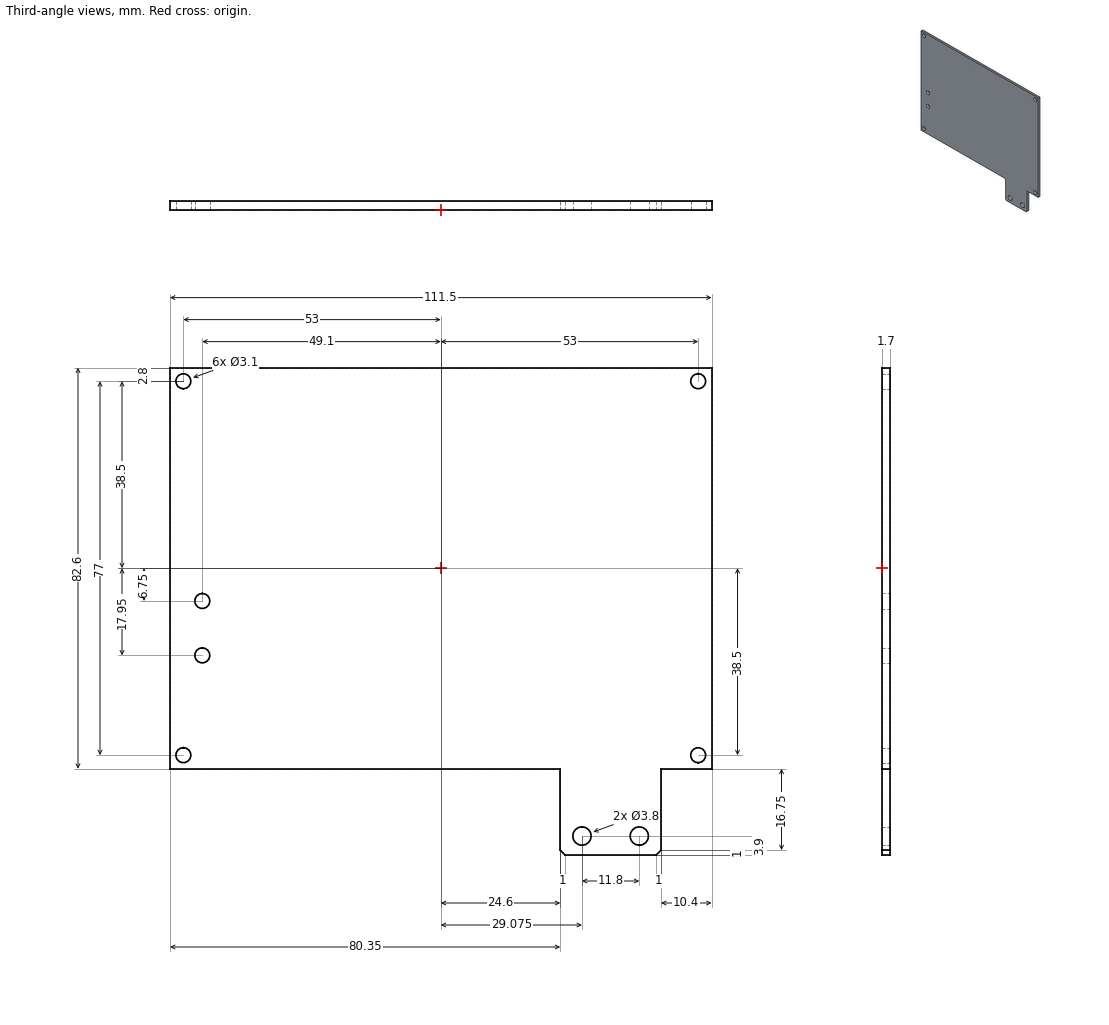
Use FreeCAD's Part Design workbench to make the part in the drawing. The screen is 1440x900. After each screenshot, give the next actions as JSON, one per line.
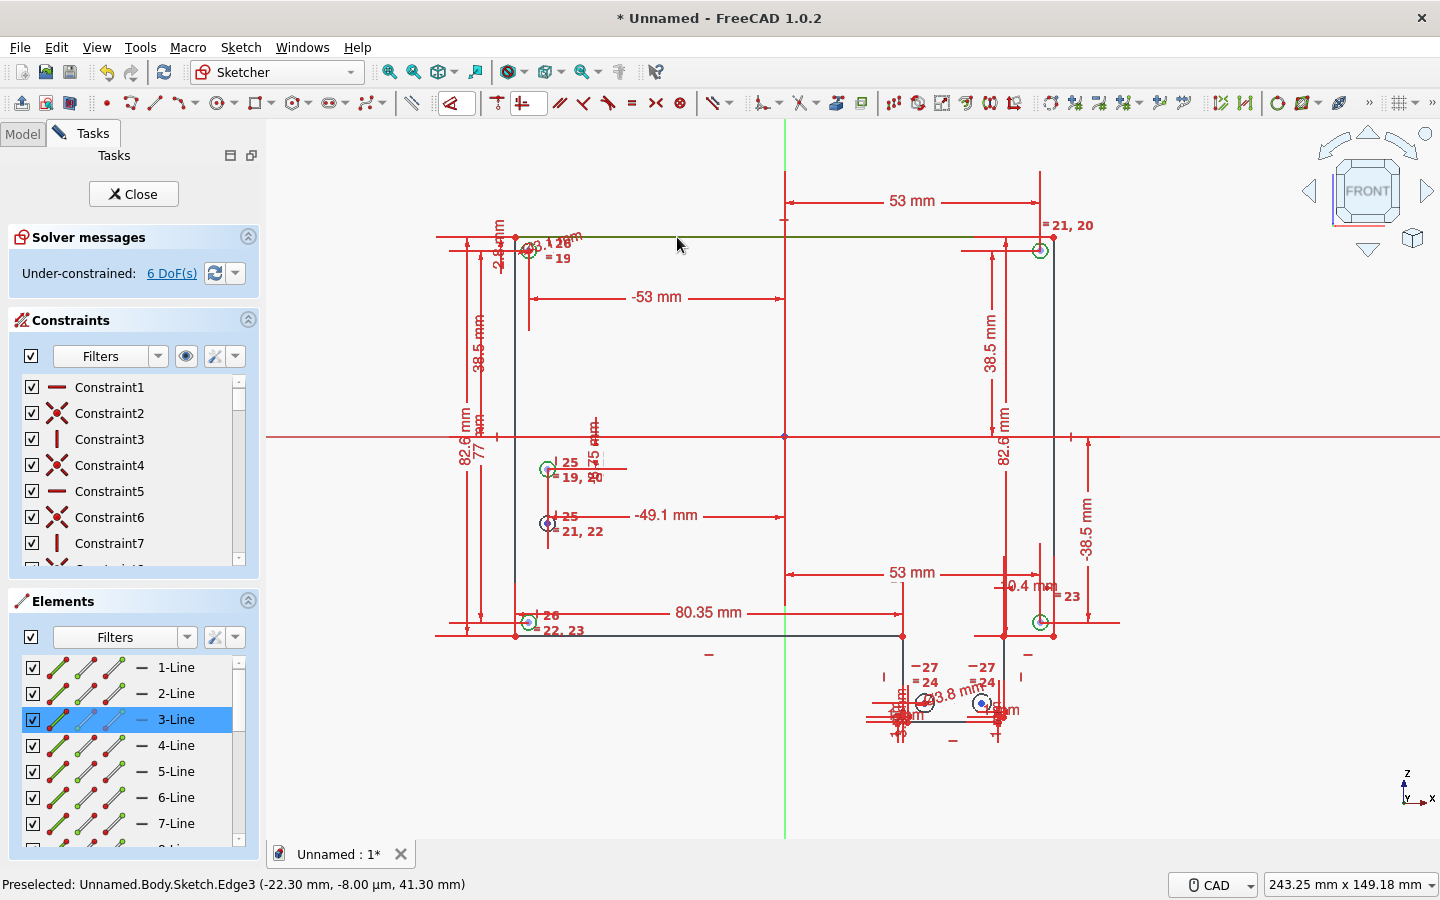
{"action": "left_click", "coordinate": [470, 104]}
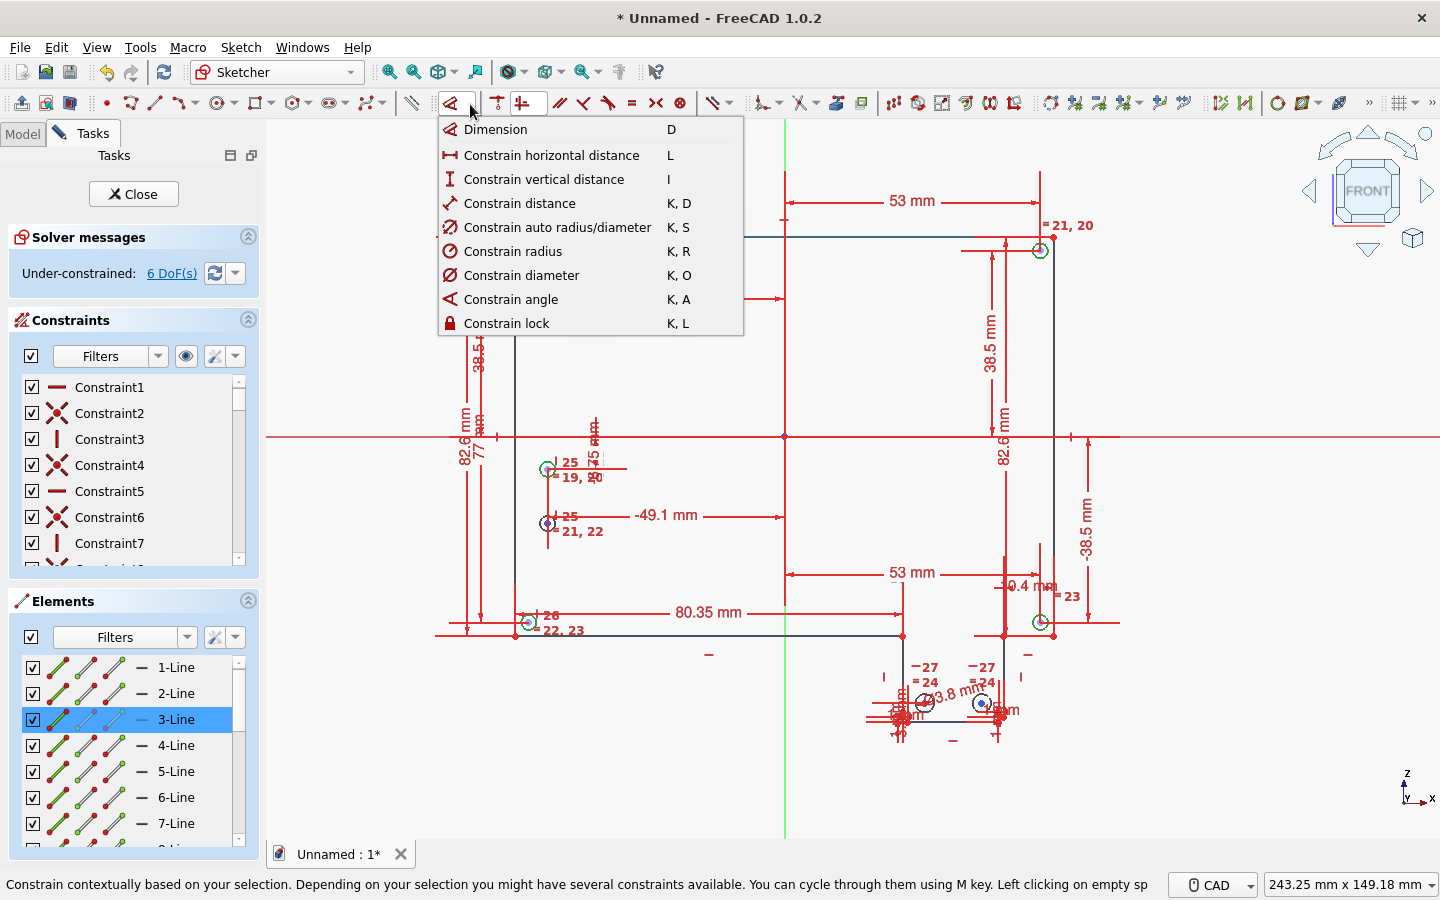
{"action": "left_click", "coordinate": [591, 155]}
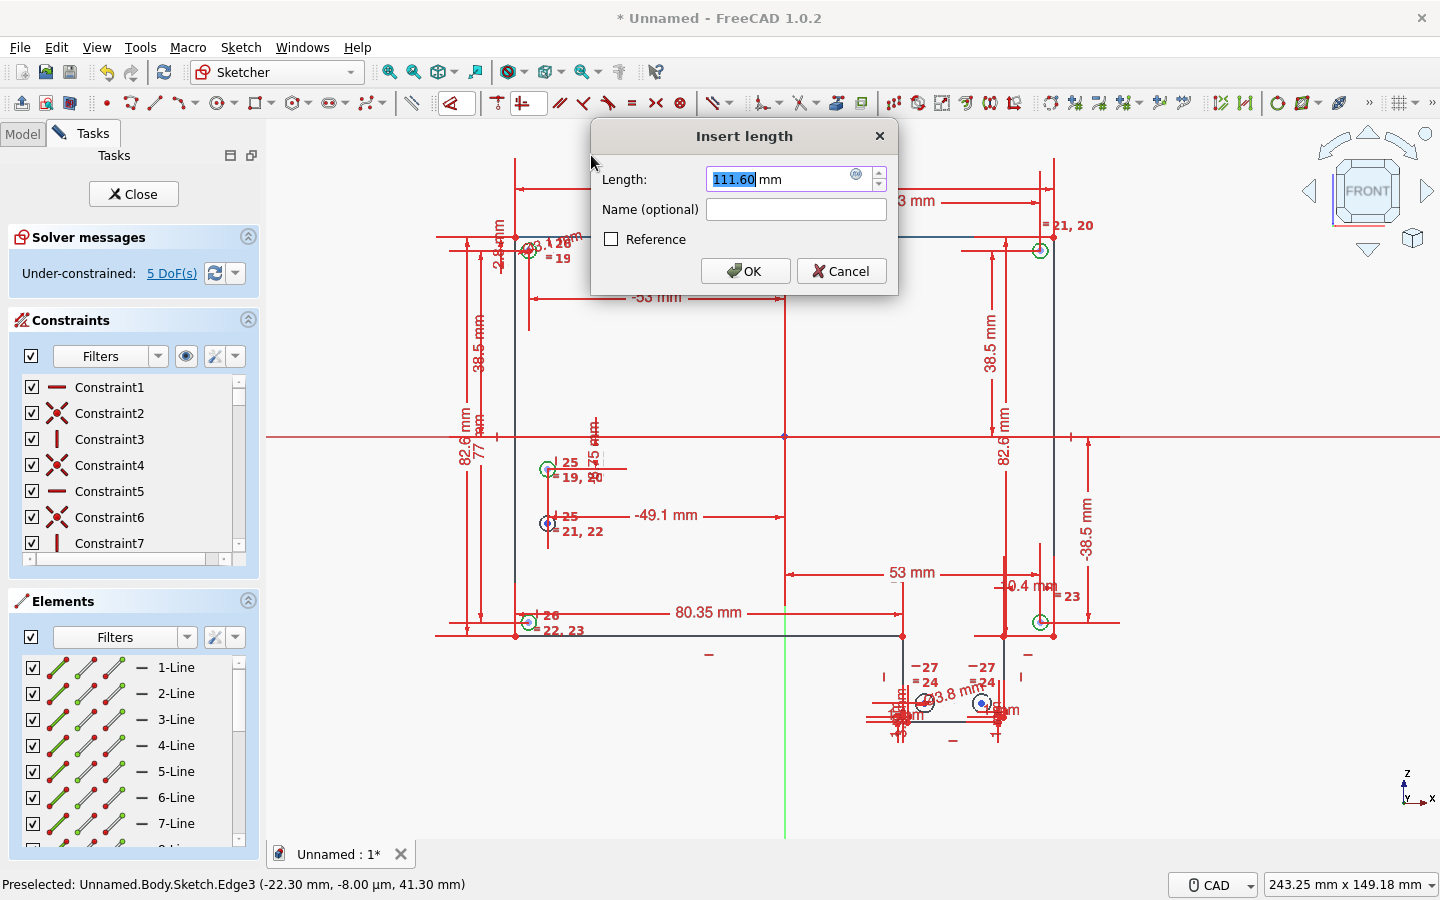
{"action": "type", "text": "111.5"}
{"action": "key", "text": "Return"}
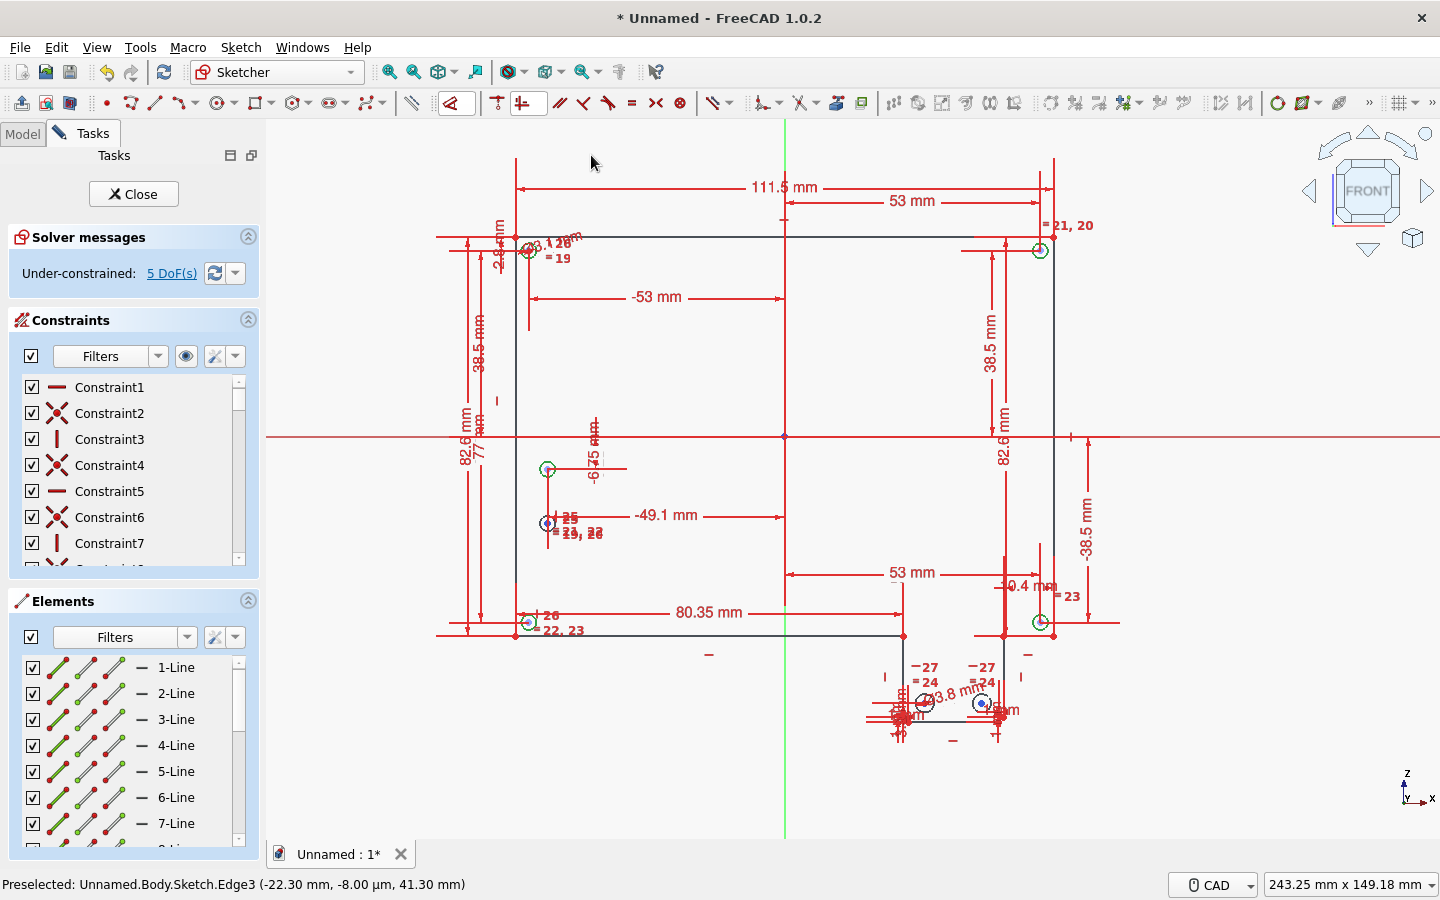
{"action": "left_click", "coordinate": [1004, 660]}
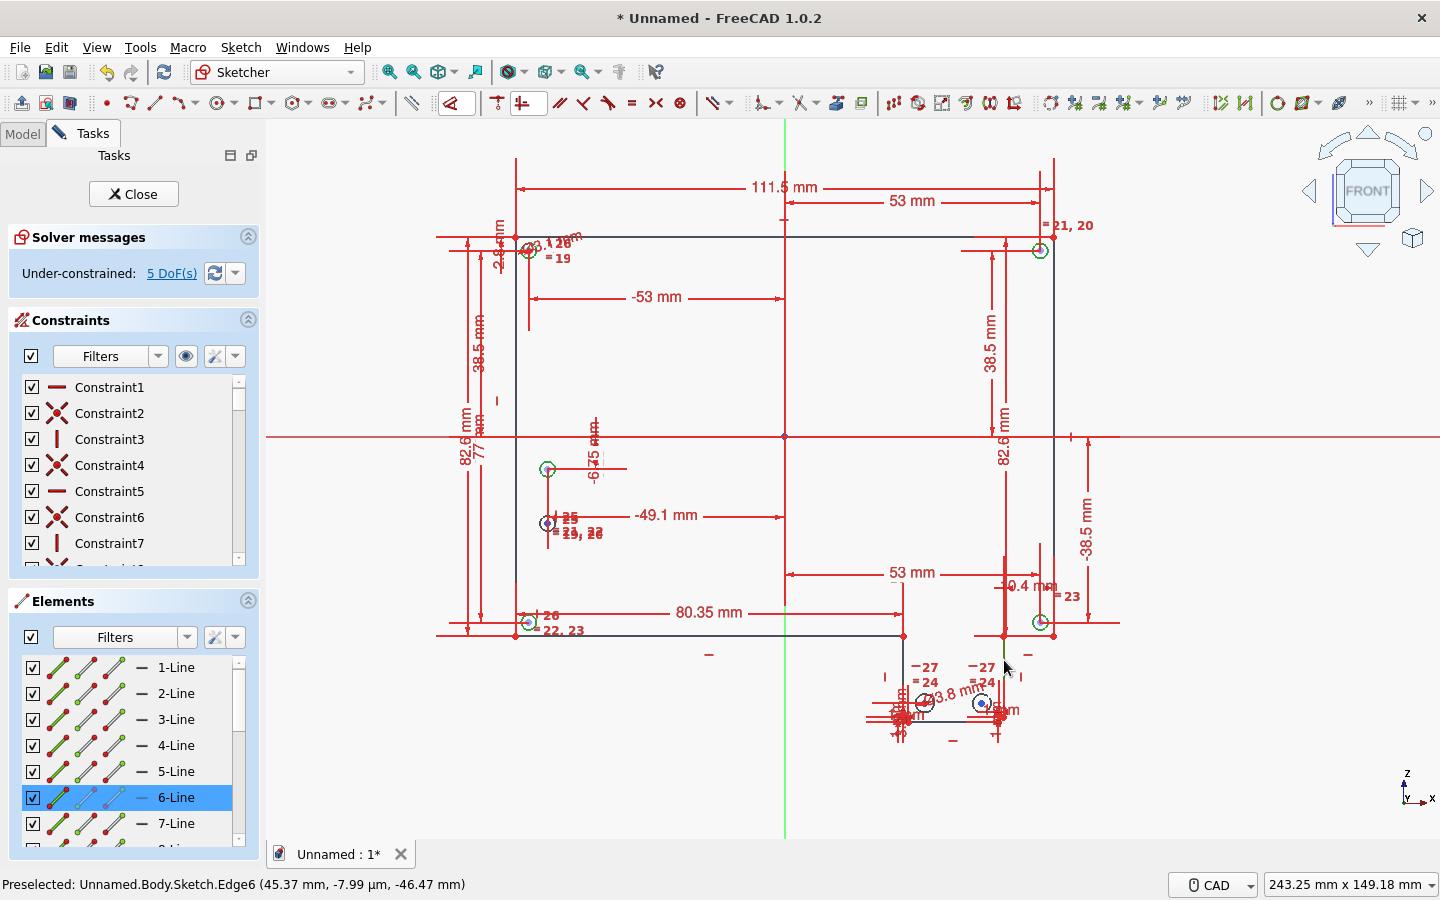
{"action": "left_click", "coordinate": [470, 104]}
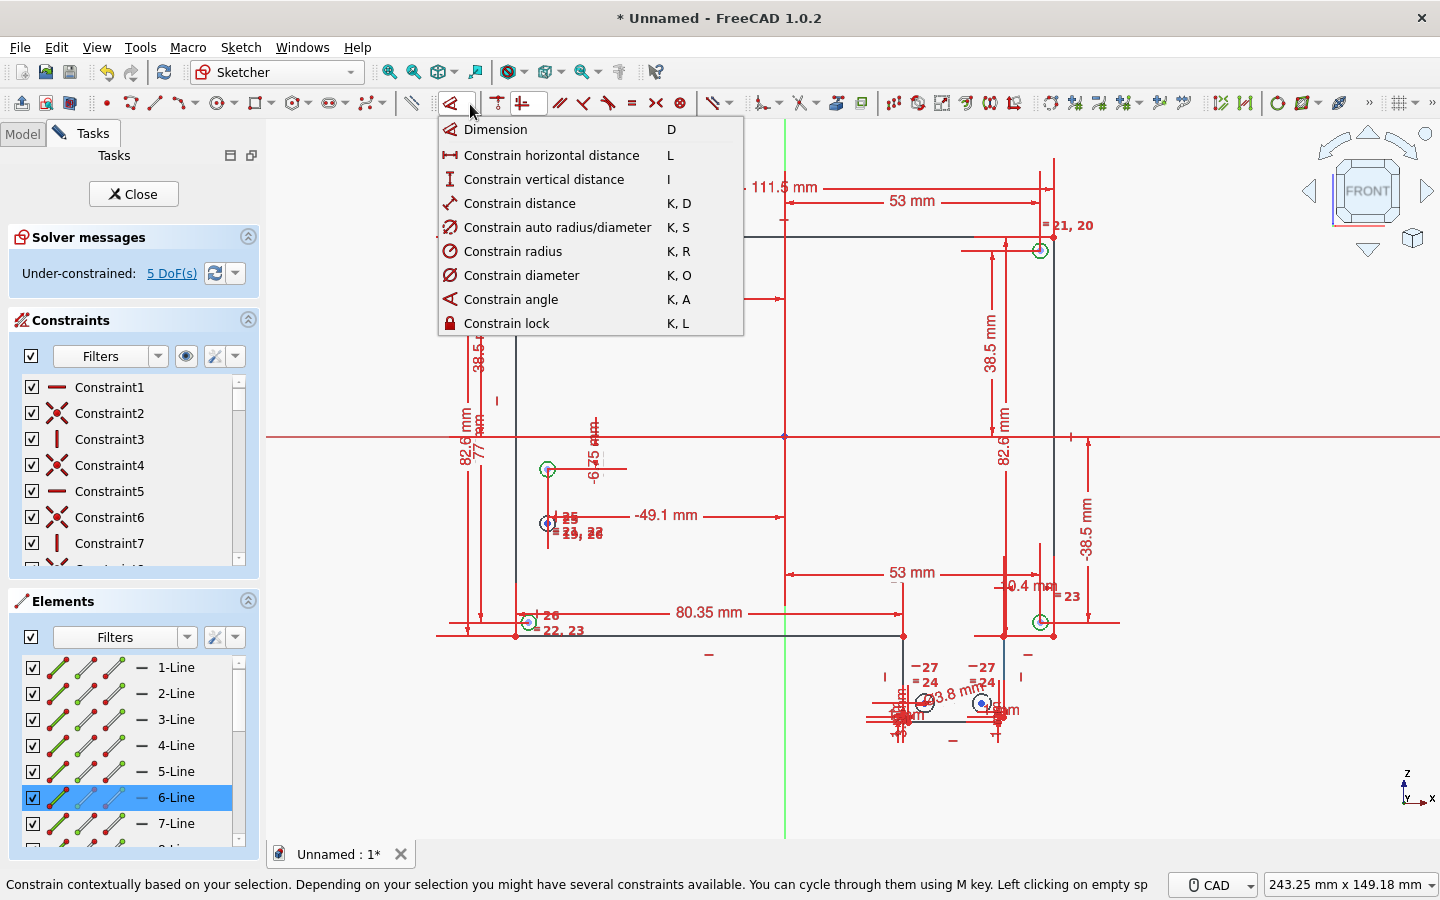
{"action": "left_click", "coordinate": [591, 179]}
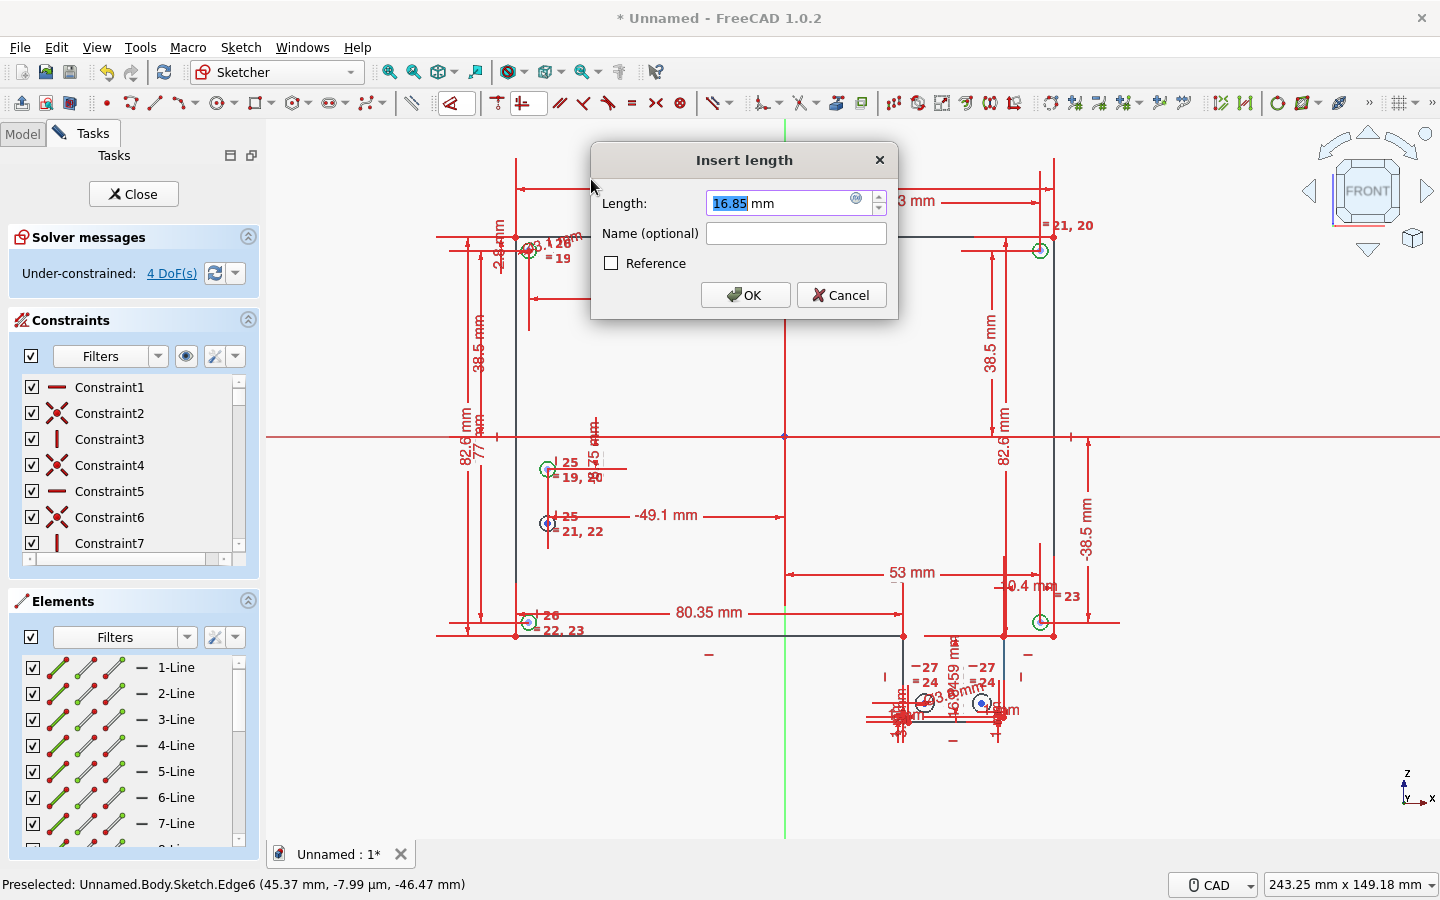
{"action": "type", "text": "16.75"}
{"action": "key", "text": "Return"}